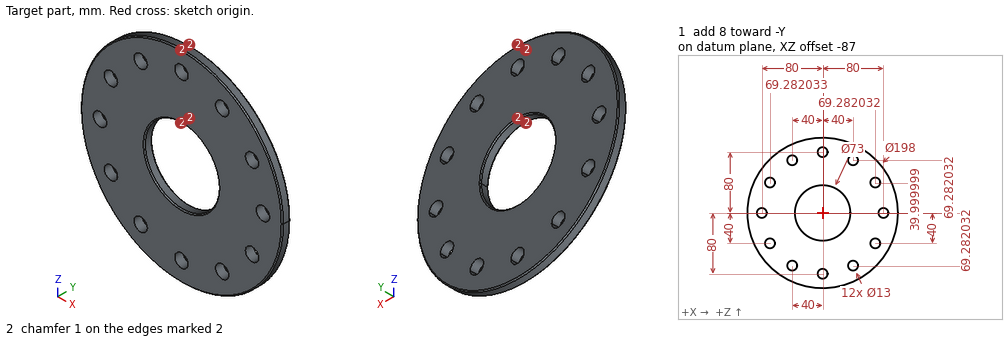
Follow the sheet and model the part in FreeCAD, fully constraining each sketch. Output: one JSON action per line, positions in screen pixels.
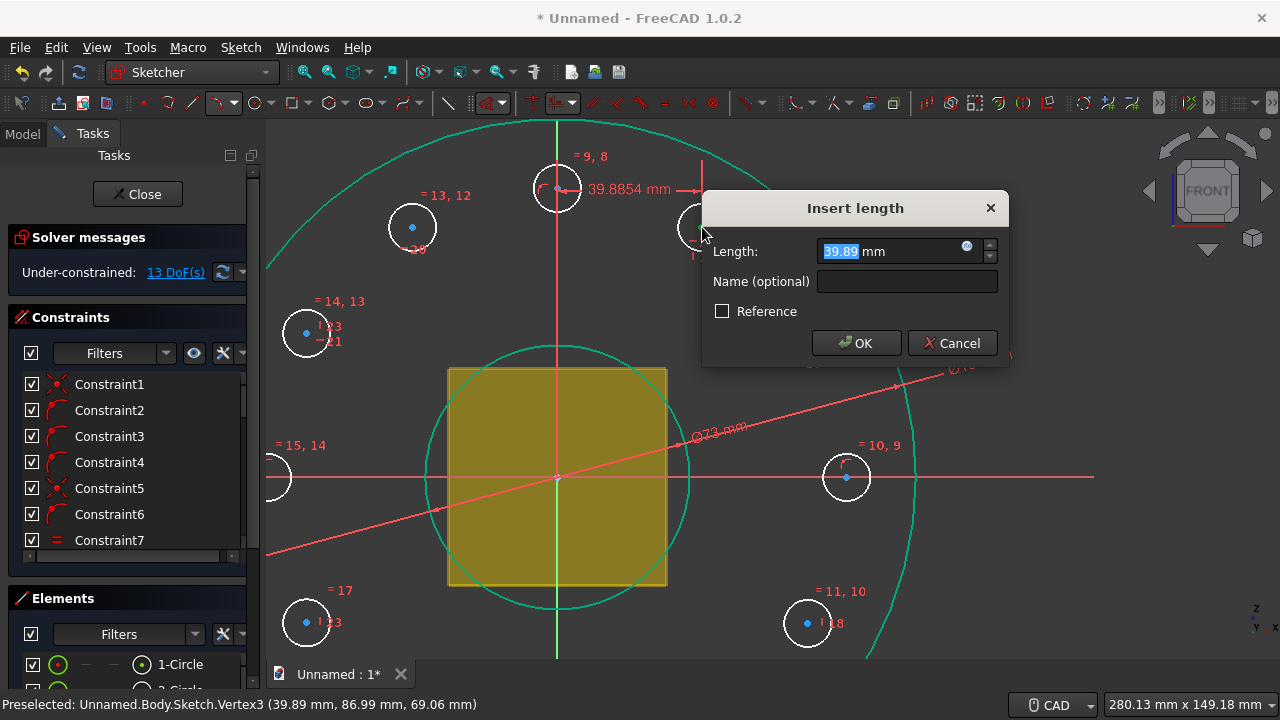
{"action": "type", "text": "40"}
{"action": "key", "text": "Return"}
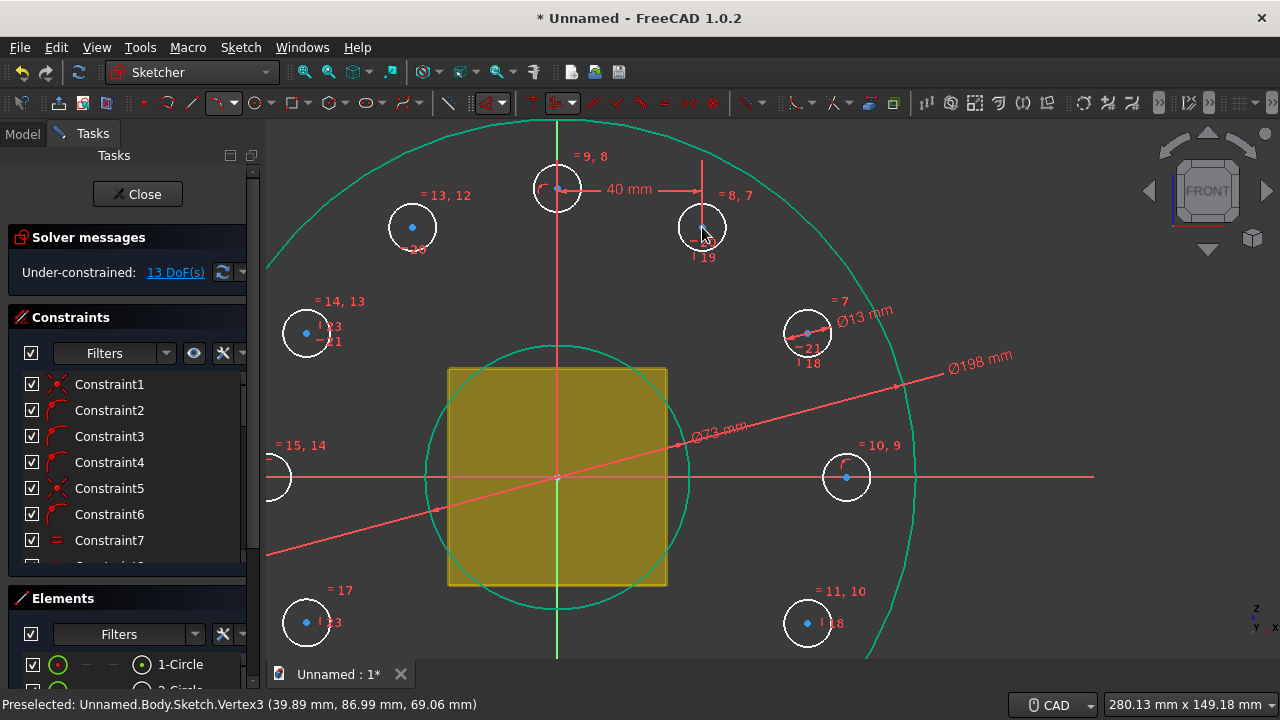
{"action": "left_click", "coordinate": [557, 188]}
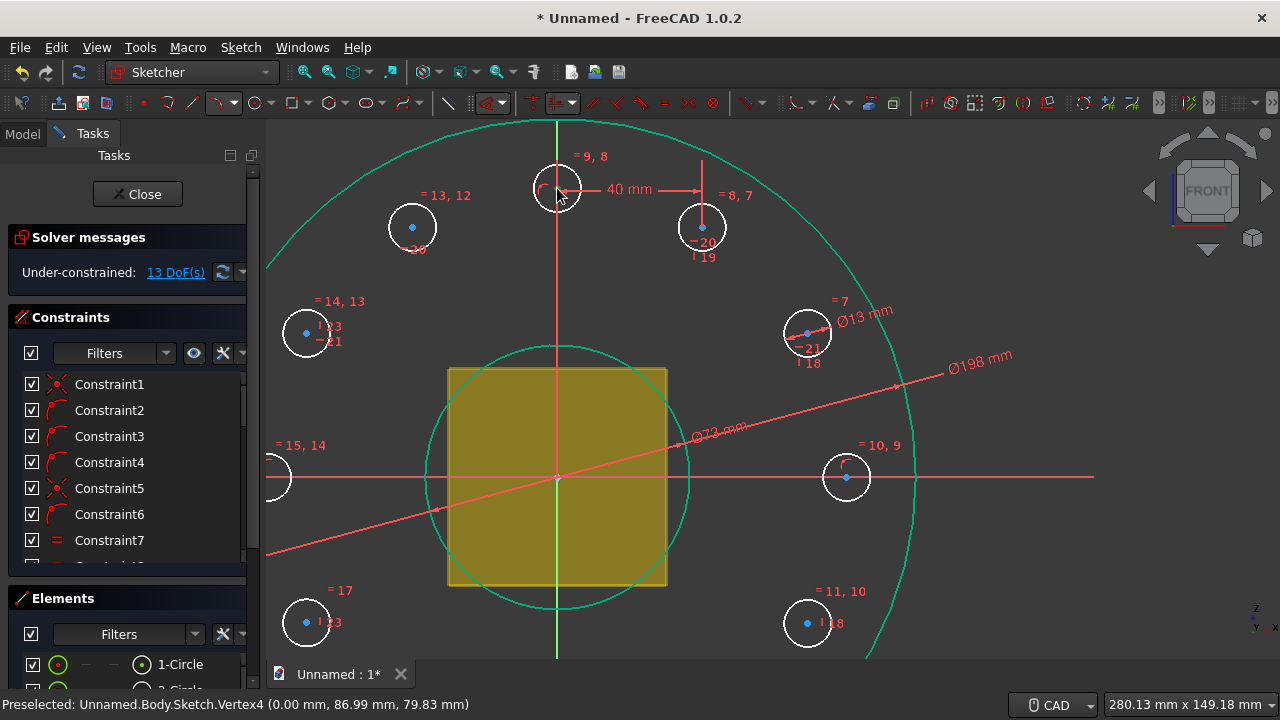
{"action": "left_click", "coordinate": [504, 104]}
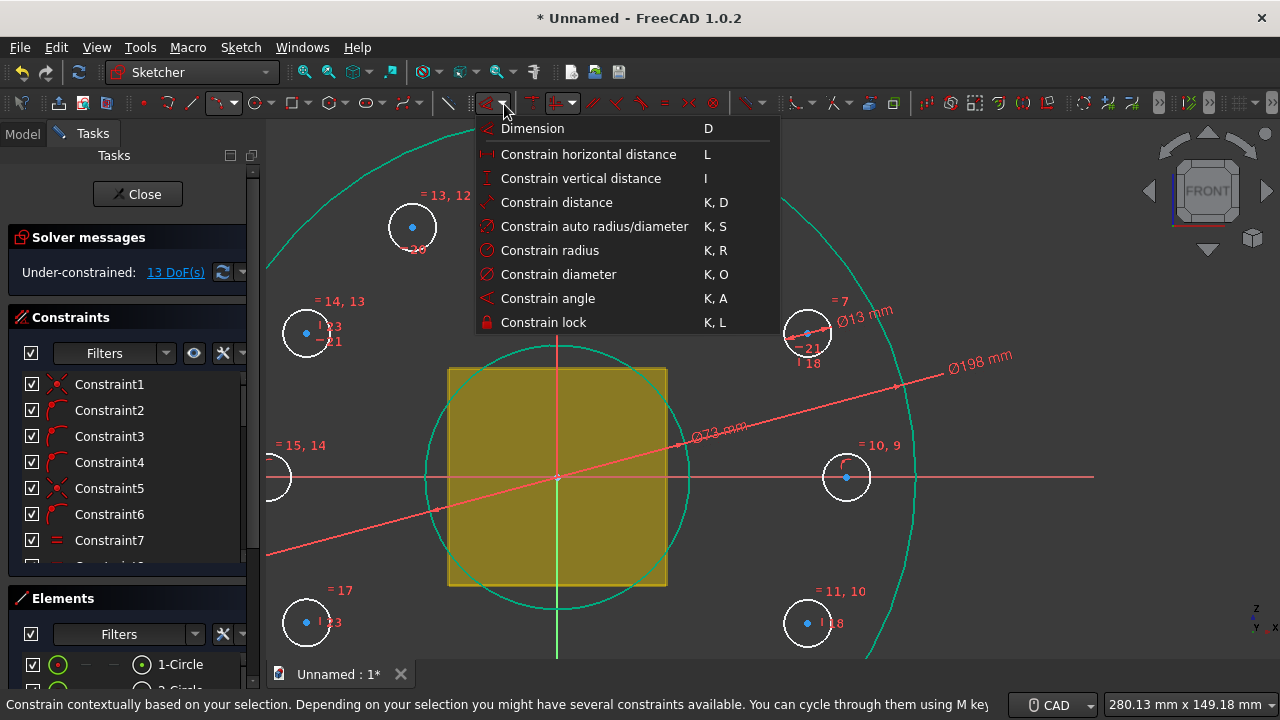
{"action": "left_click", "coordinate": [628, 178]}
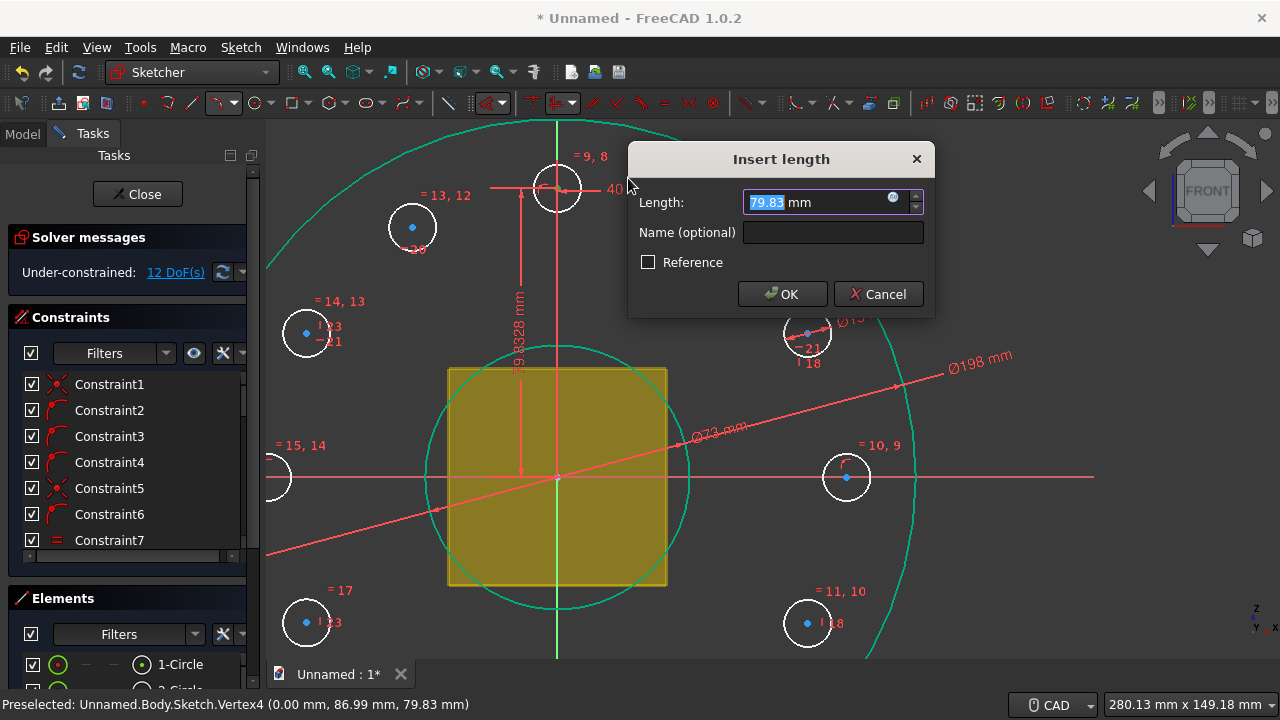
{"action": "type", "text": "80"}
{"action": "key", "text": "Return"}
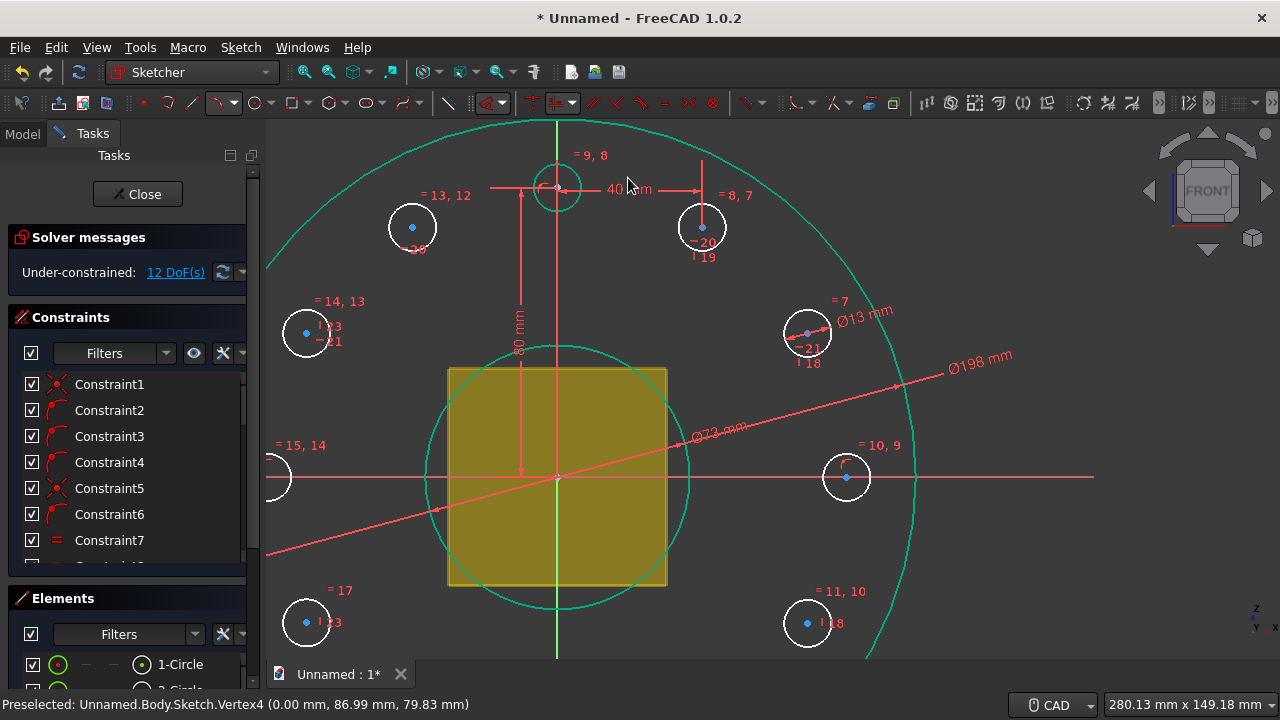
{"action": "left_click", "coordinate": [847, 477]}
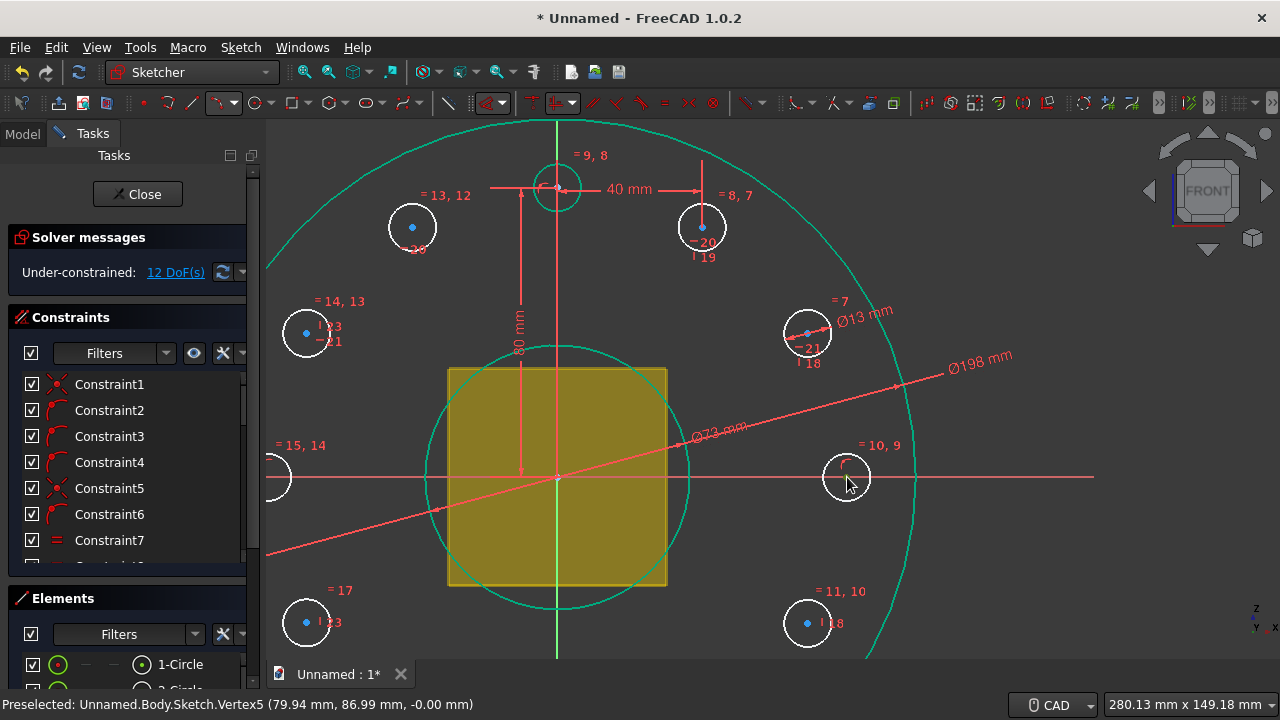
{"action": "key", "text": "l"}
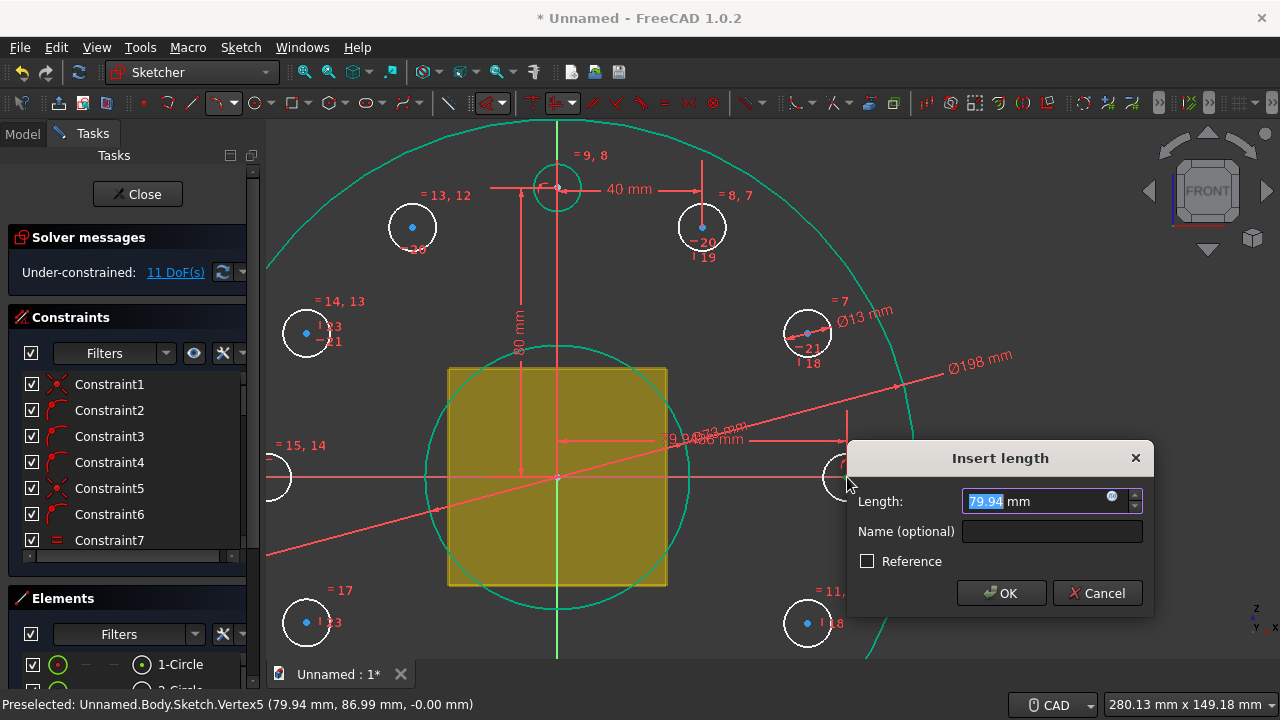
{"action": "type", "text": "80"}
{"action": "key", "text": "Return"}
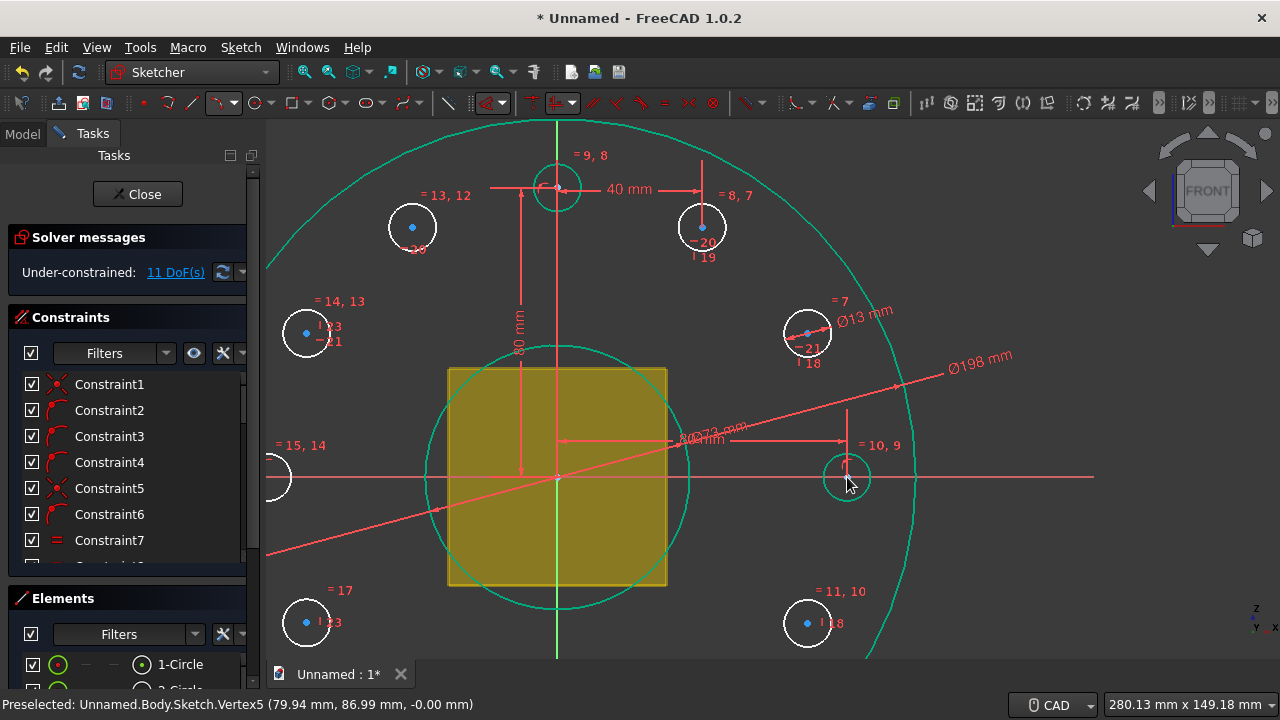
{"action": "left_click", "coordinate": [808, 623]}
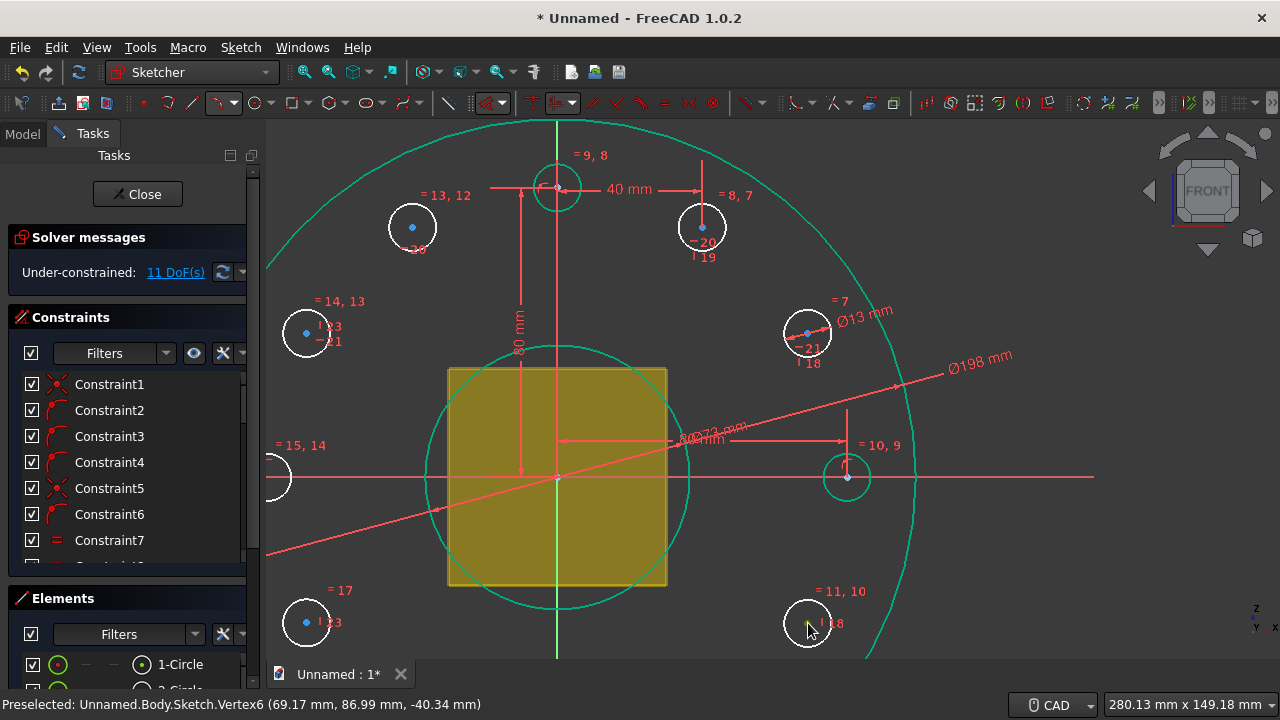
{"action": "key", "text": "i"}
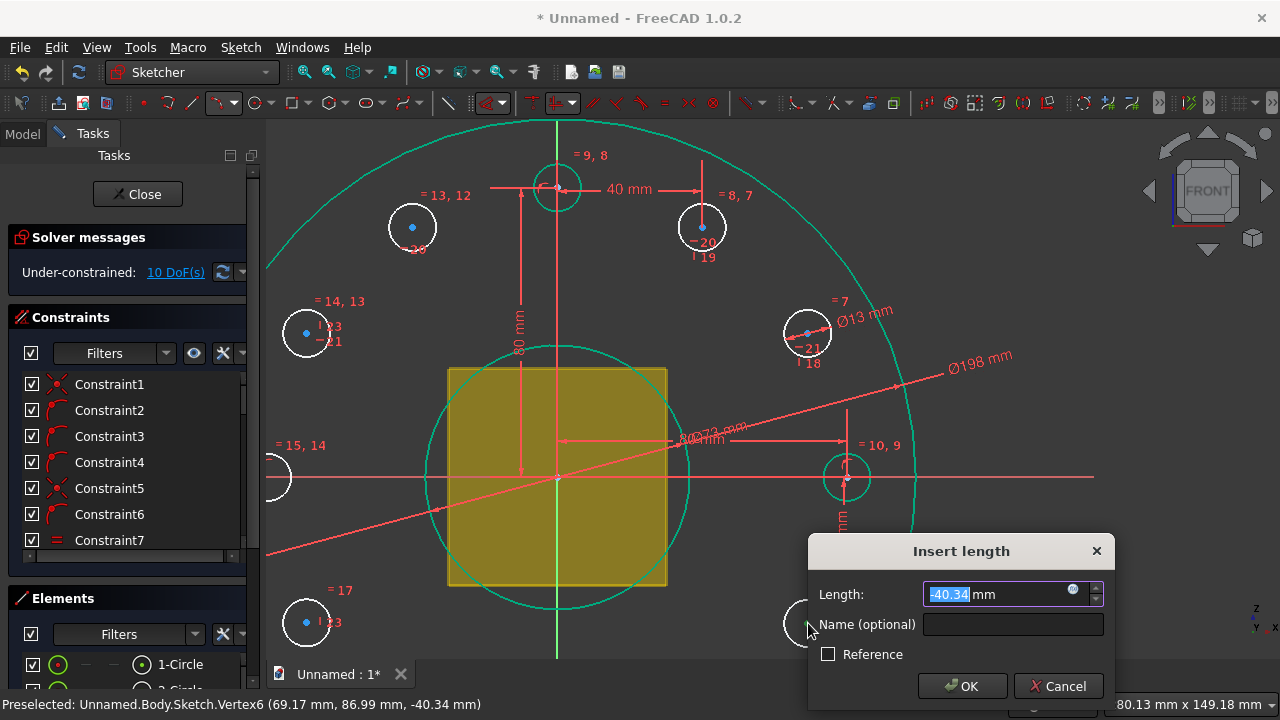
{"action": "type", "text": "-40"}
{"action": "key", "text": "Return"}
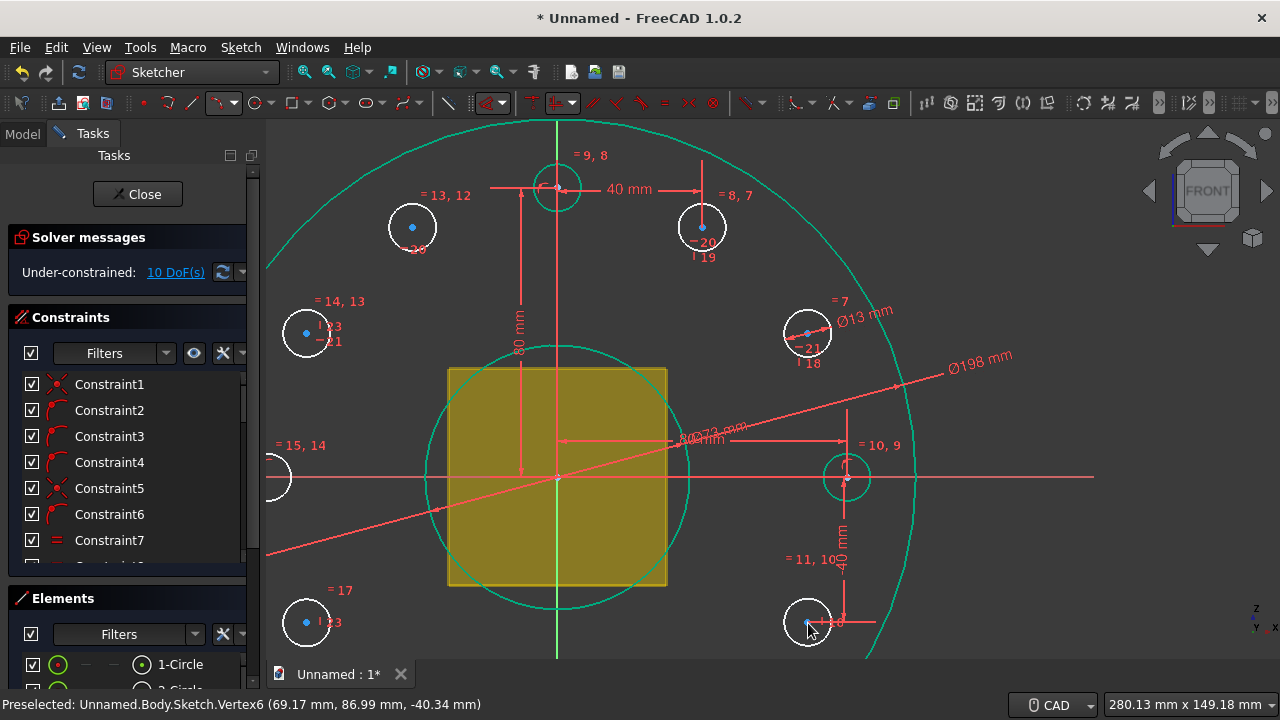
{"action": "left_click", "coordinate": [413, 227]}